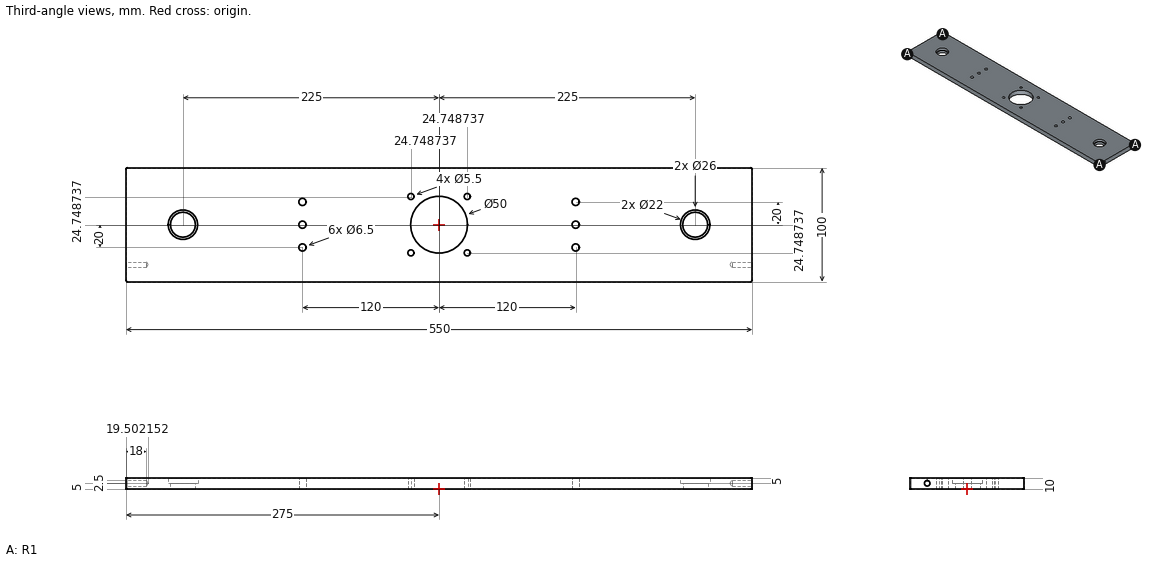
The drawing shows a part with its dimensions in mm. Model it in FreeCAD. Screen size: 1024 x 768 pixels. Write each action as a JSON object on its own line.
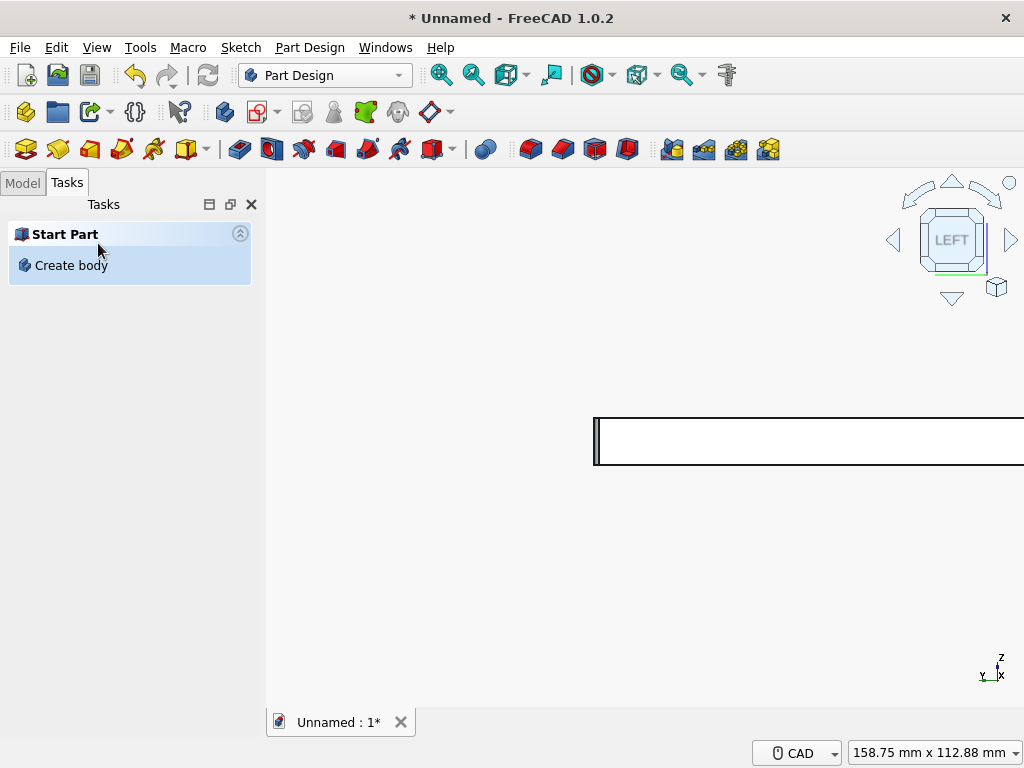
{"action": "key", "text": "v f"}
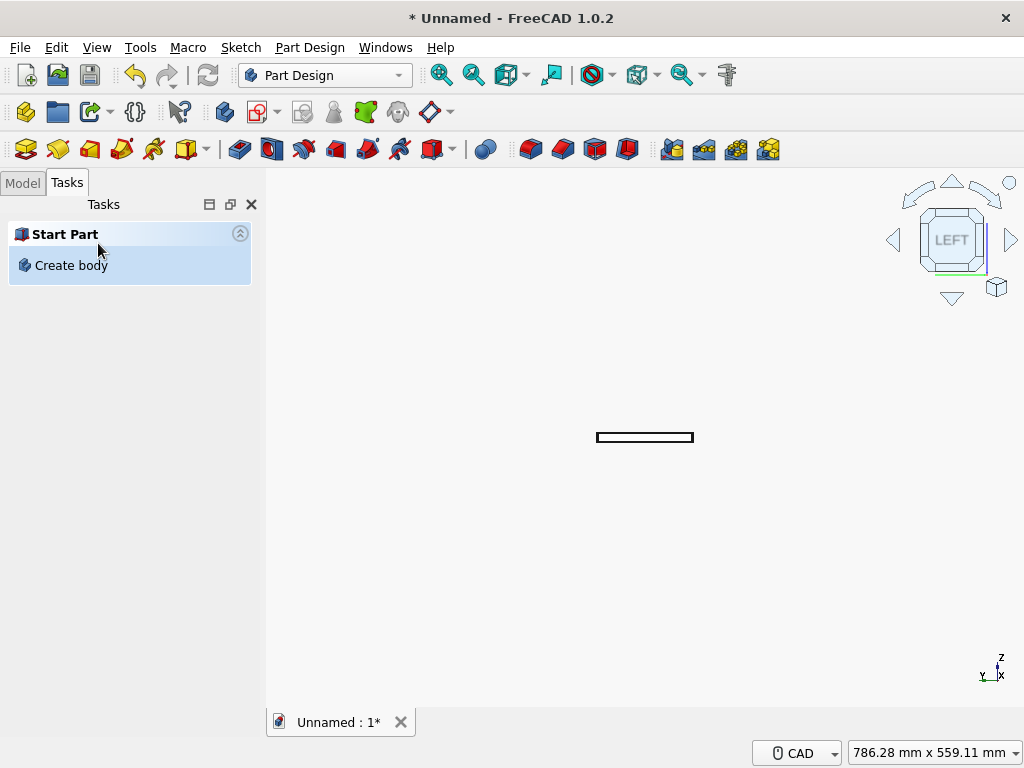
{"action": "left_click", "coordinate": [23, 182]}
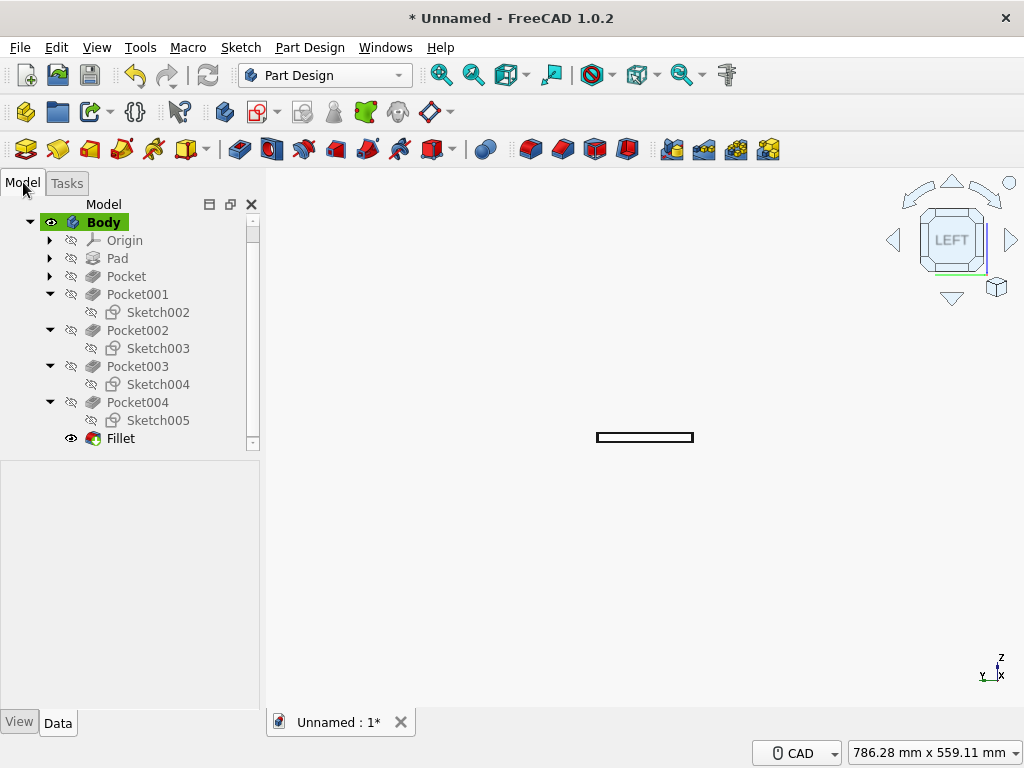
{"action": "left_click", "coordinate": [50, 240]}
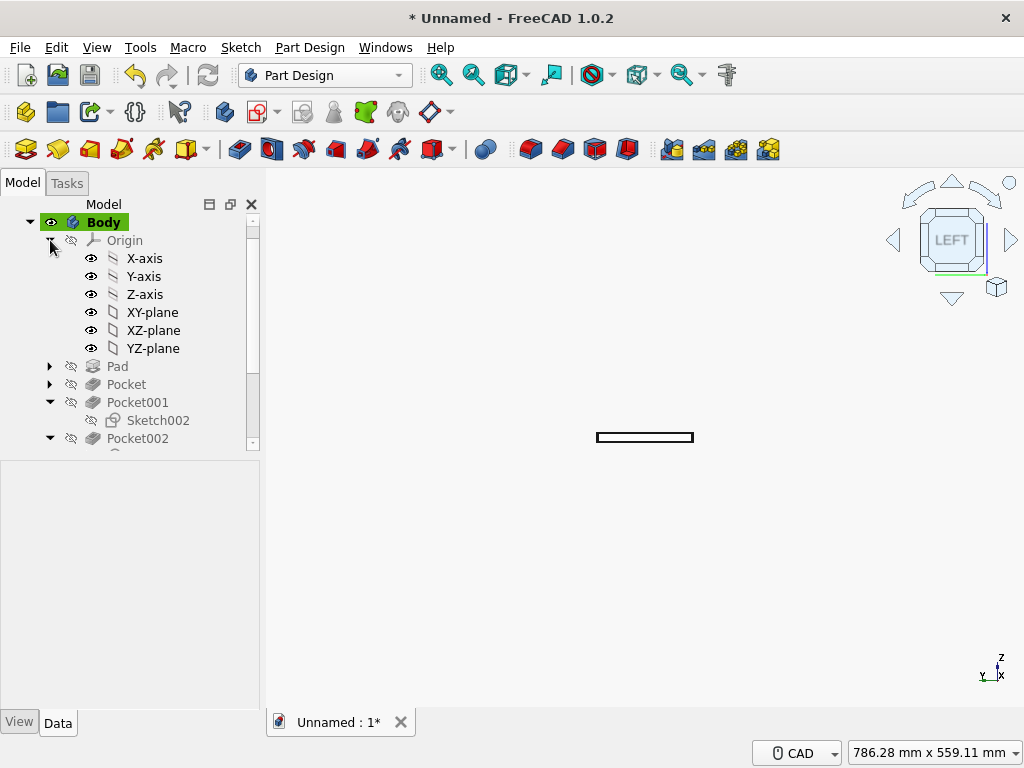
{"action": "left_click", "coordinate": [136, 330]}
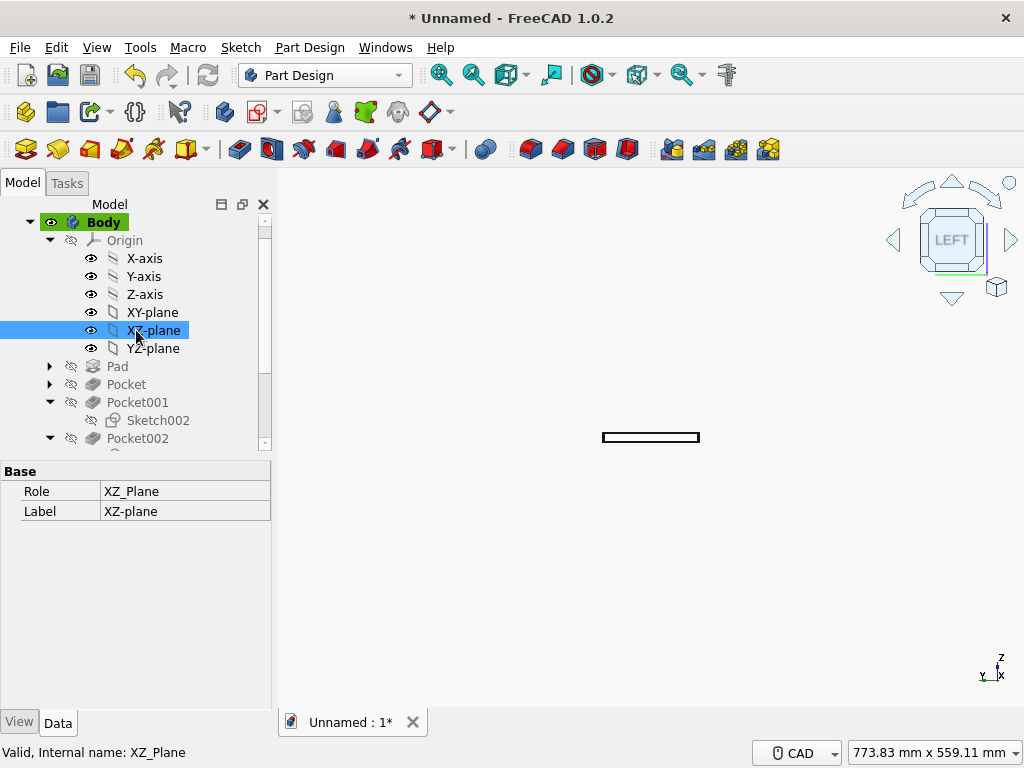
{"action": "left_click", "coordinate": [430, 112]}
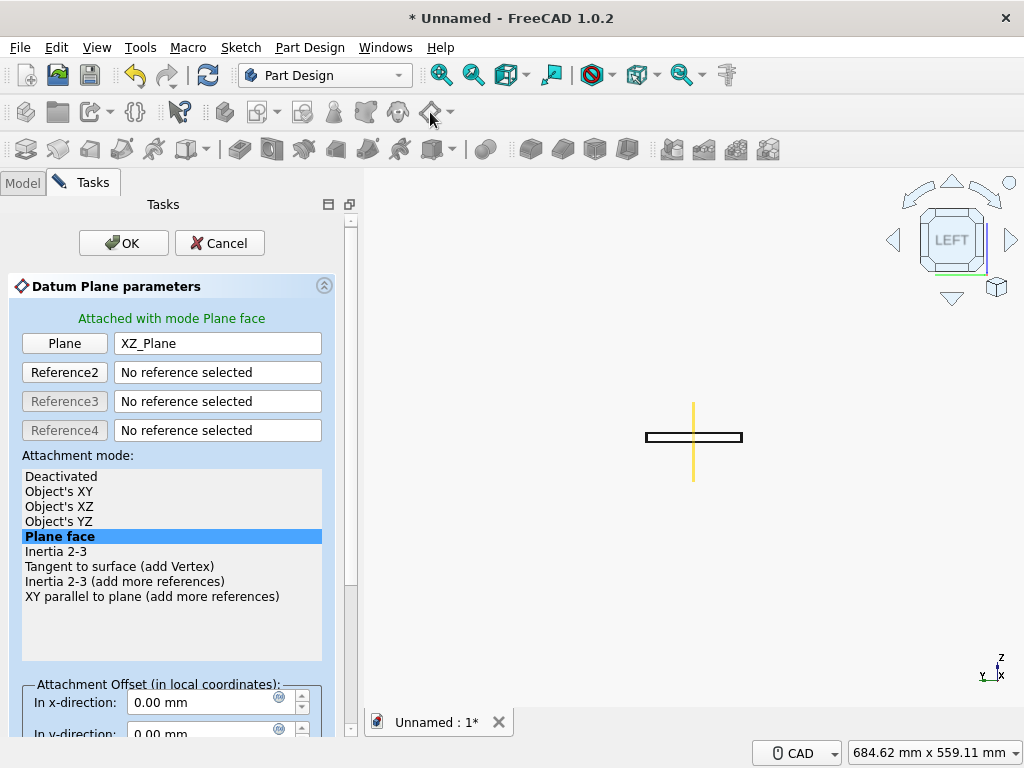
{"action": "scroll", "coordinate": [351, 475], "scroll_direction": "down", "scroll_amount": 2}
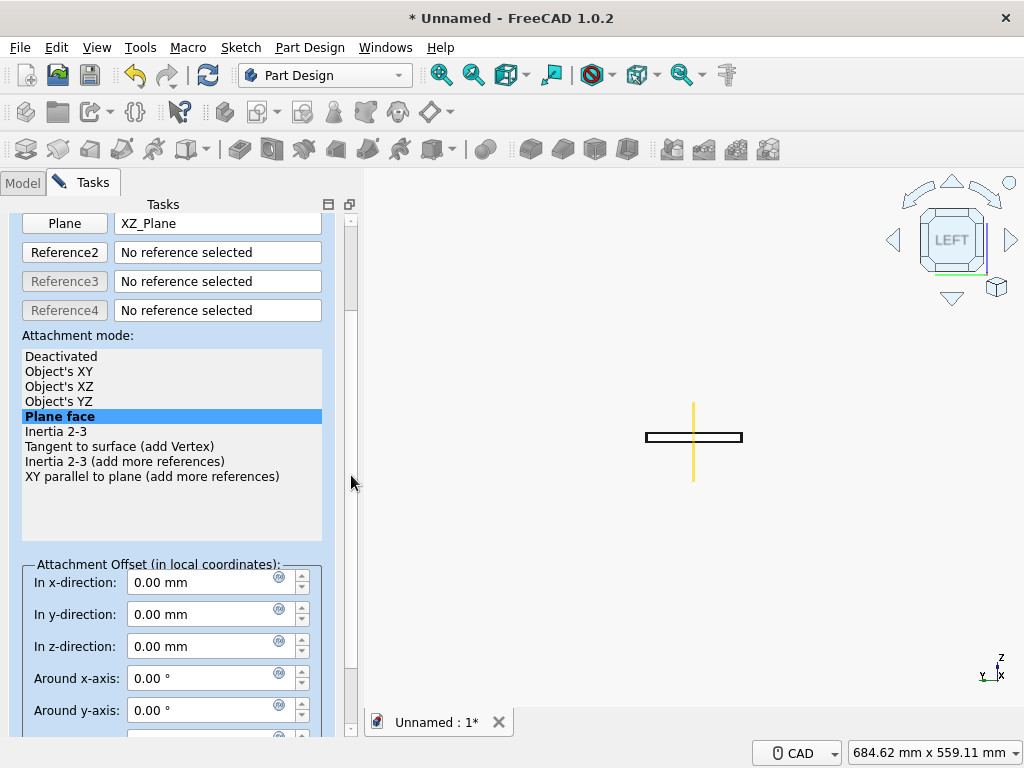
{"action": "triple_click", "coordinate": [210, 646]}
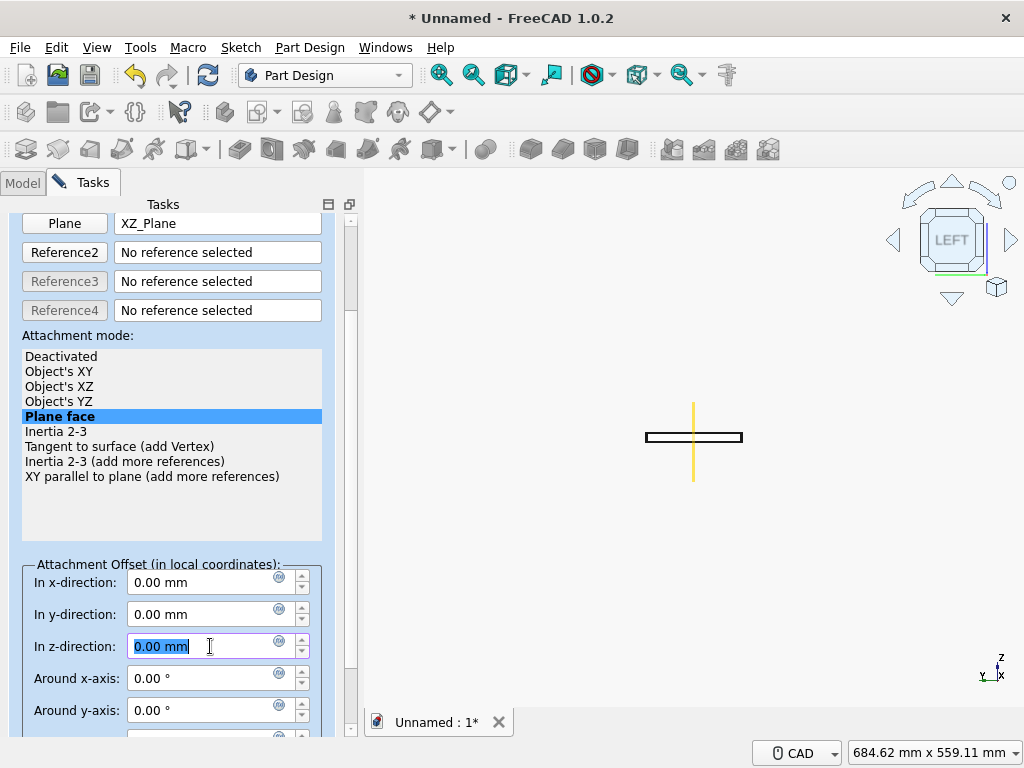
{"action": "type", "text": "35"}
{"action": "key", "text": "Tab"}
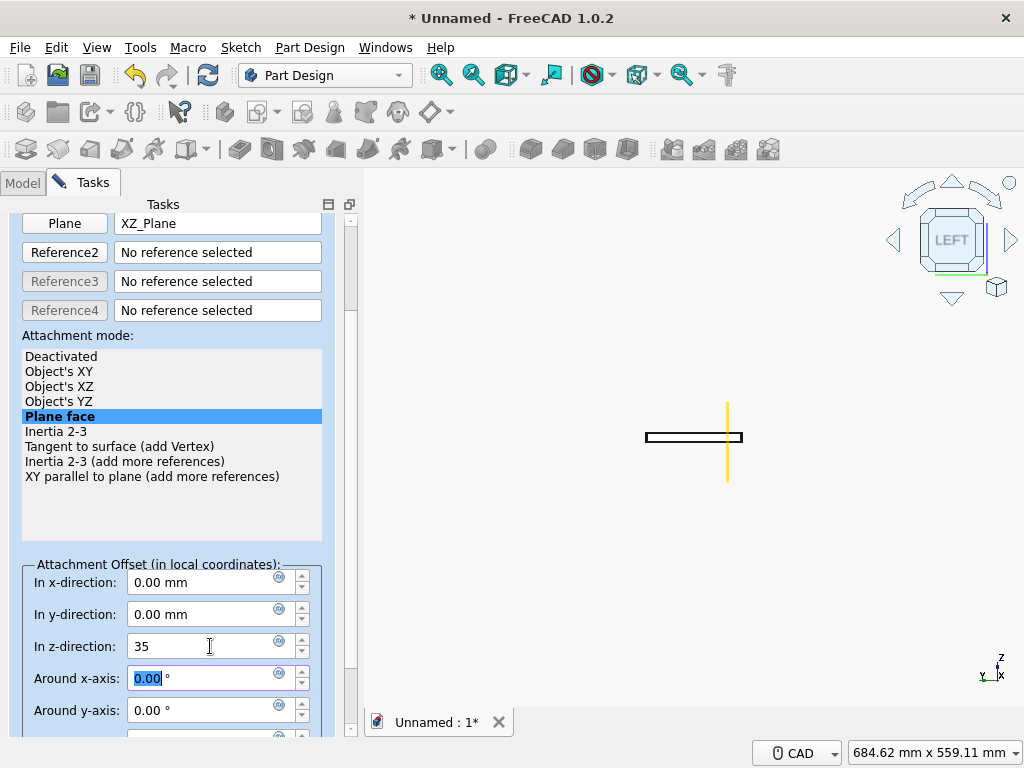
{"action": "scroll", "coordinate": [351, 475], "scroll_direction": "up", "scroll_amount": 3}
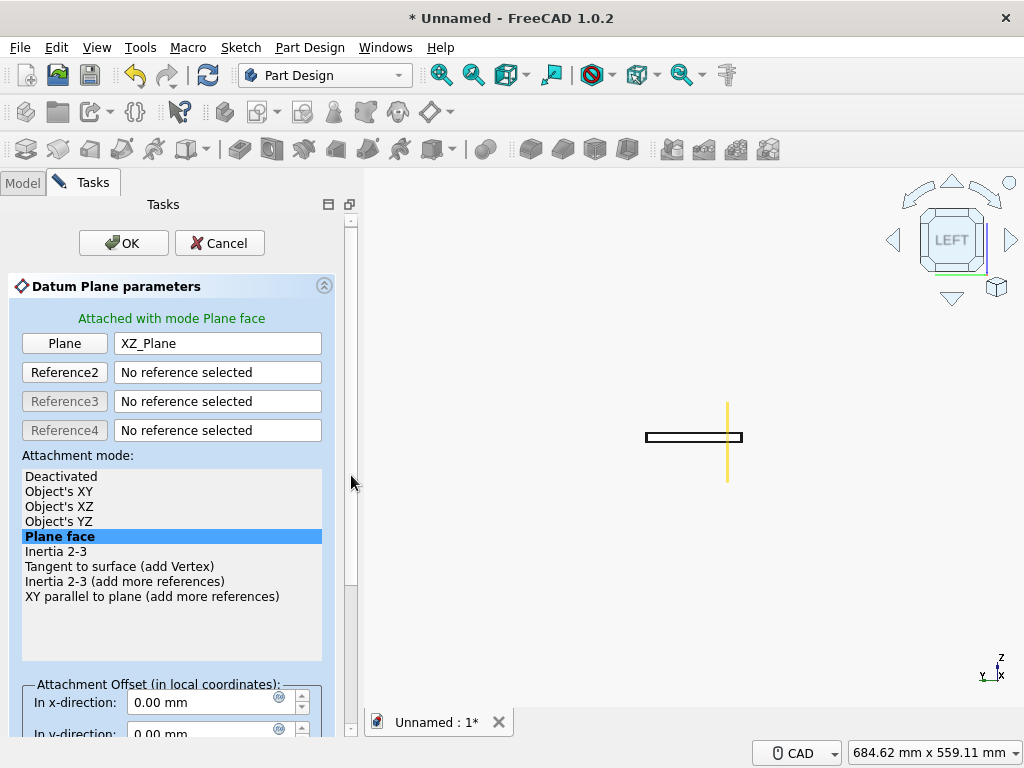
{"action": "left_click", "coordinate": [124, 243]}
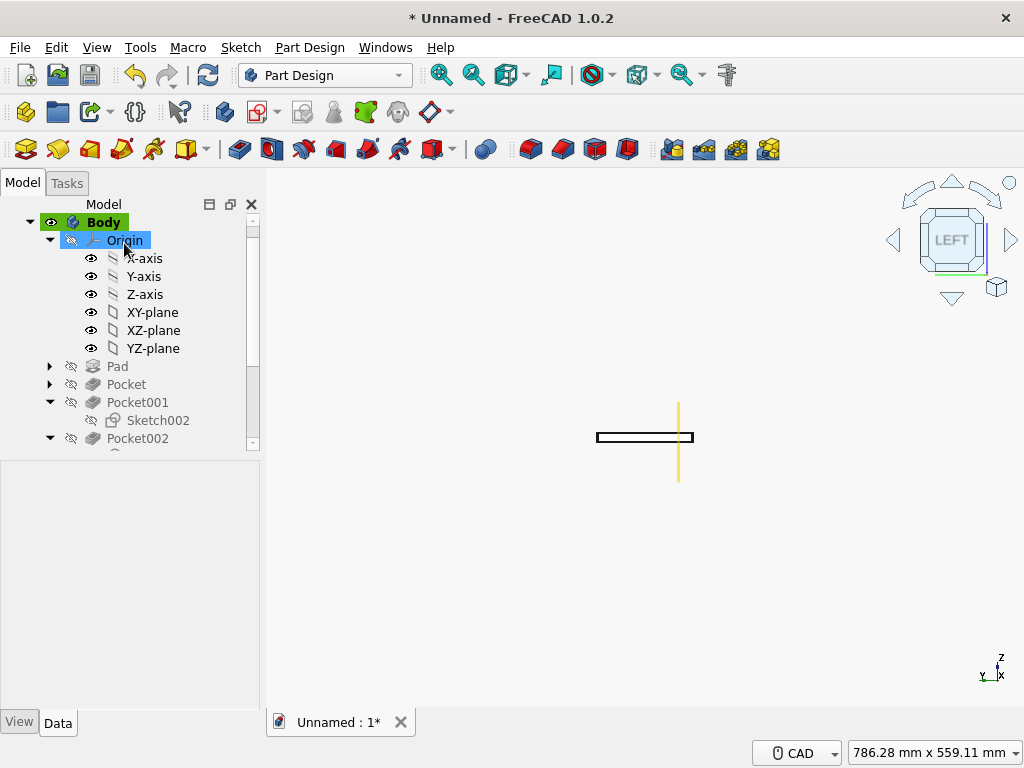
{"action": "scroll", "coordinate": [120, 326], "scroll_direction": "down", "scroll_amount": 3}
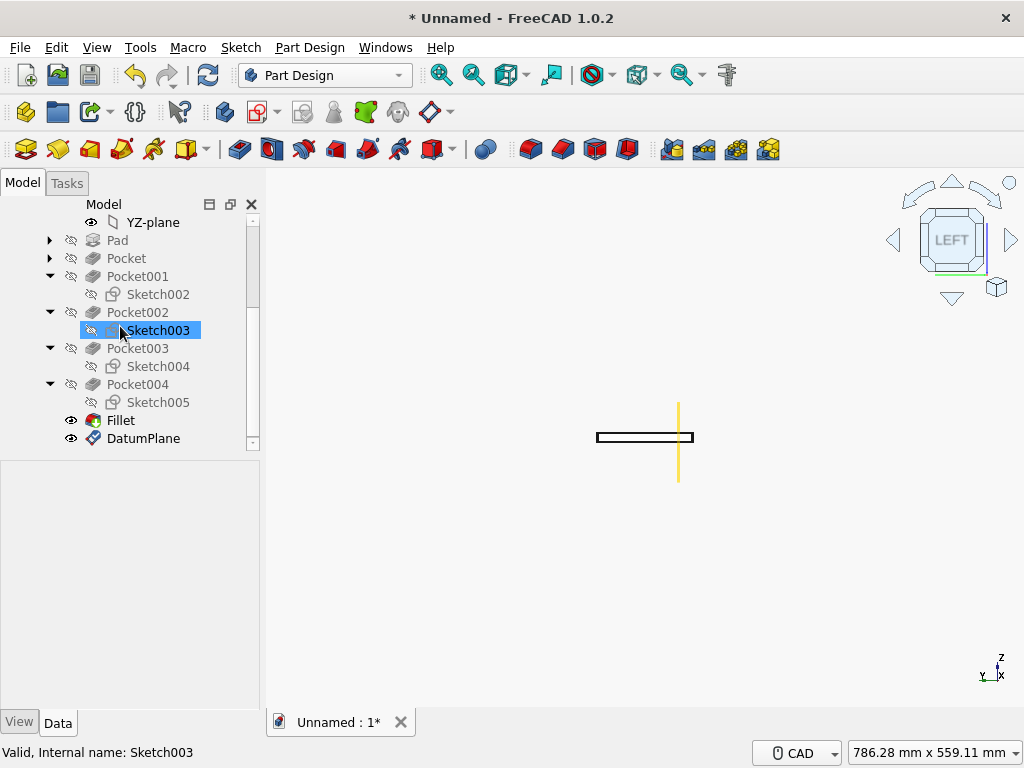
{"action": "left_click", "coordinate": [116, 438]}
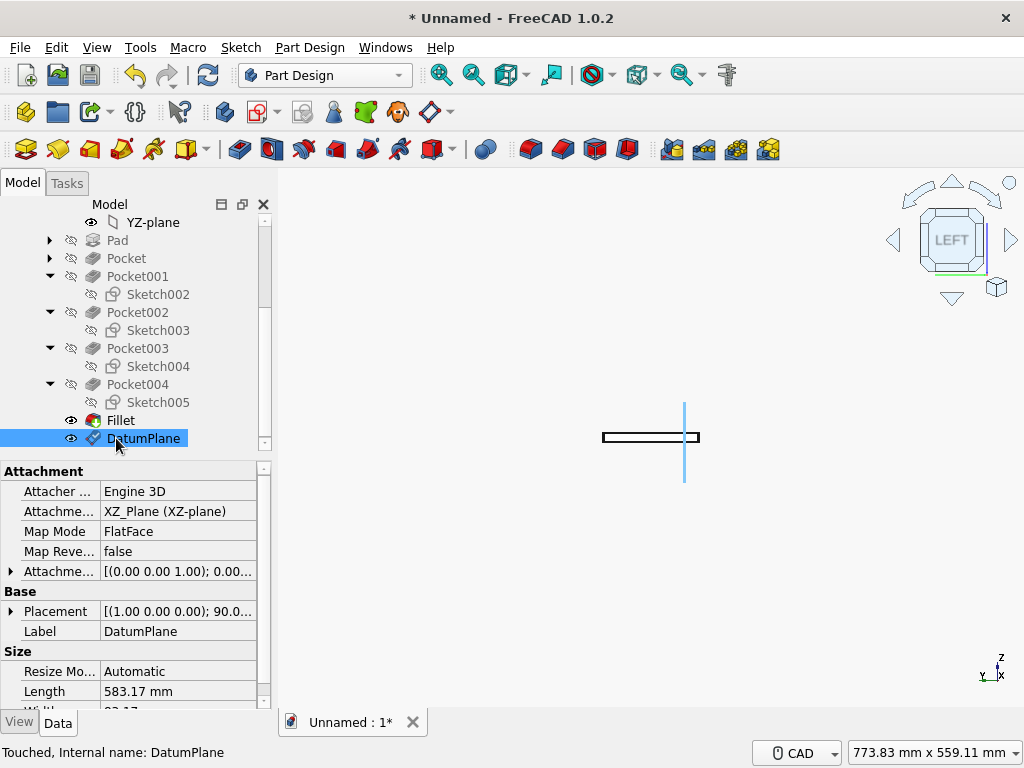
{"action": "left_click", "coordinate": [258, 112]}